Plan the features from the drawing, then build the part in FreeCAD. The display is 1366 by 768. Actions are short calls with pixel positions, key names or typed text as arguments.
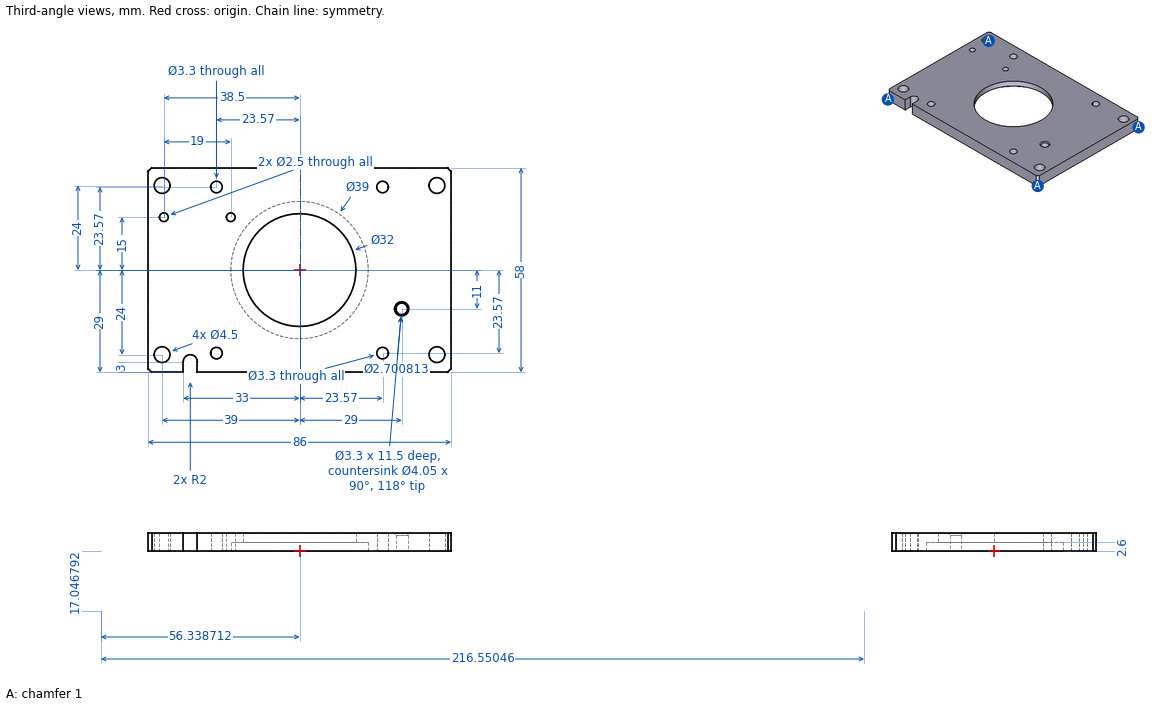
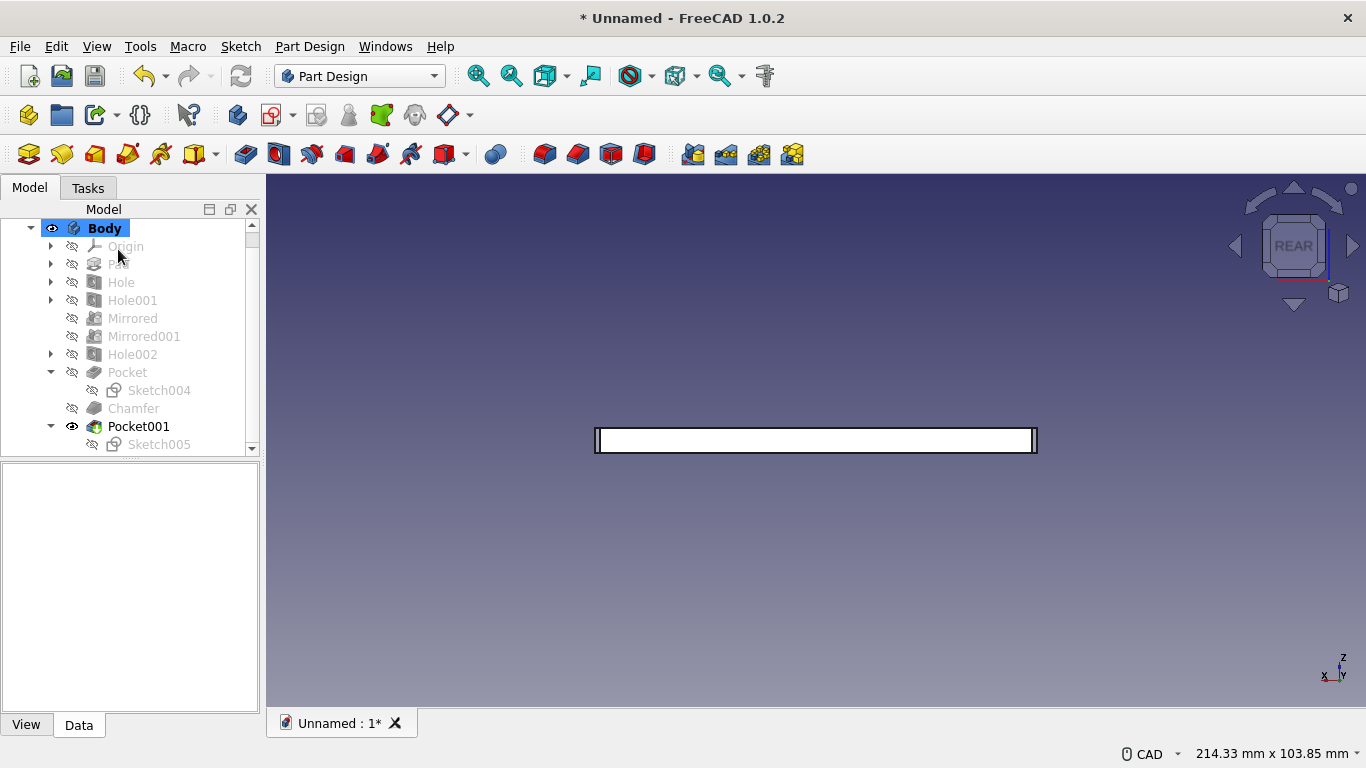
click(270, 116)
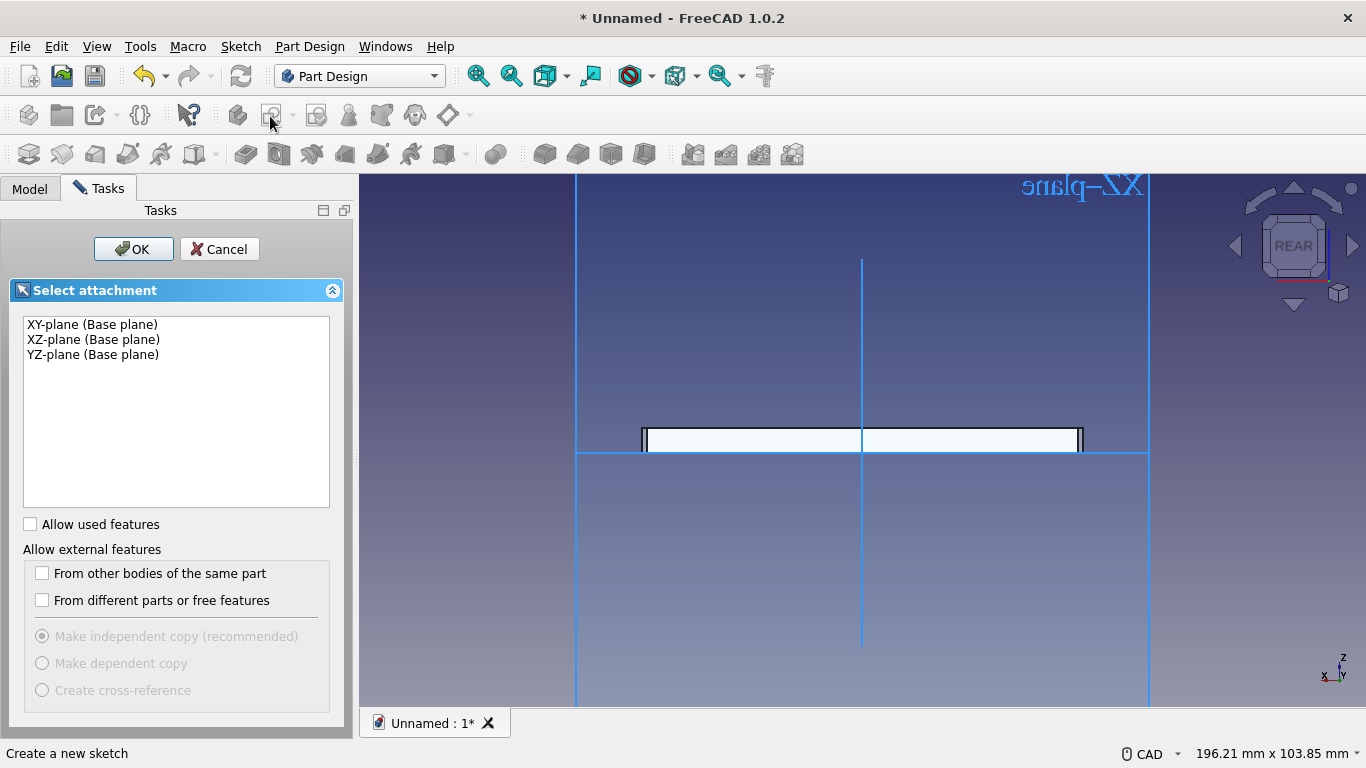
click(84, 324)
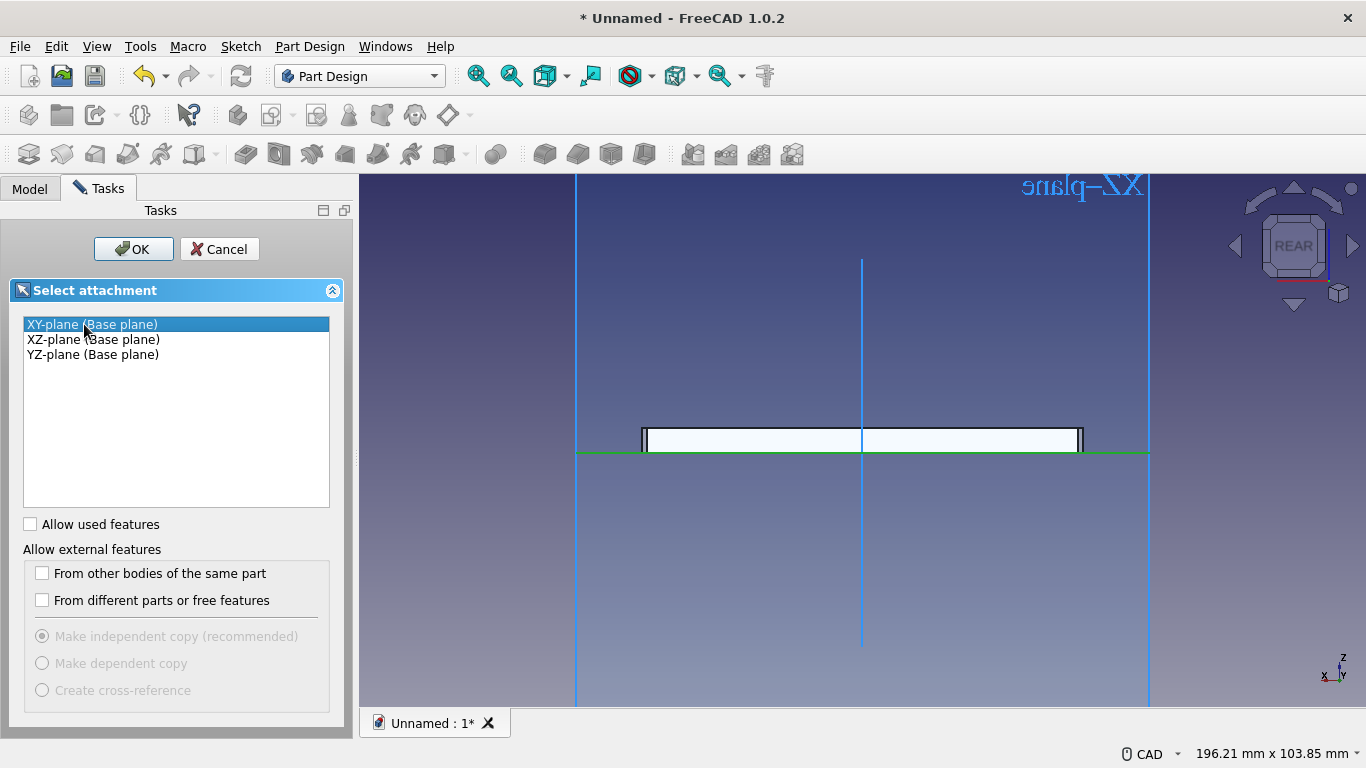
click(134, 249)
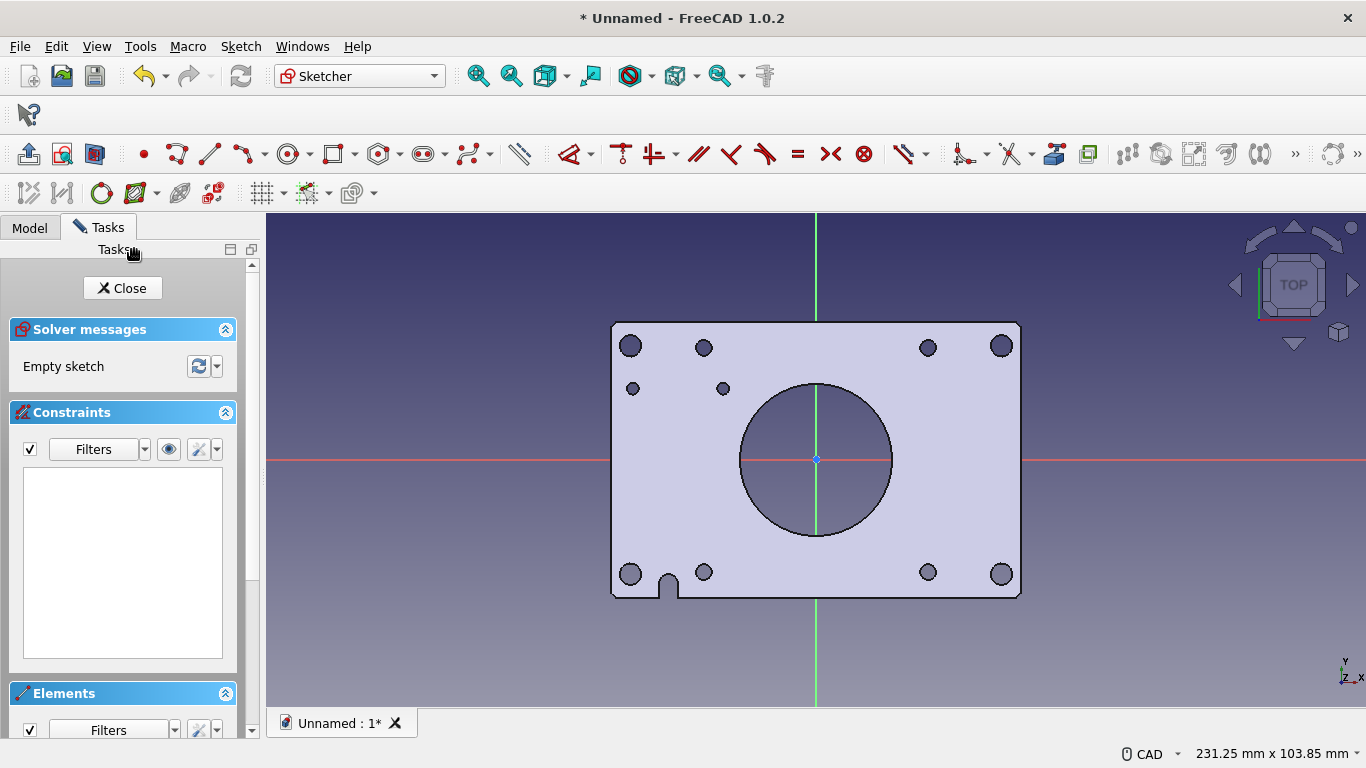
key(q)
key(s)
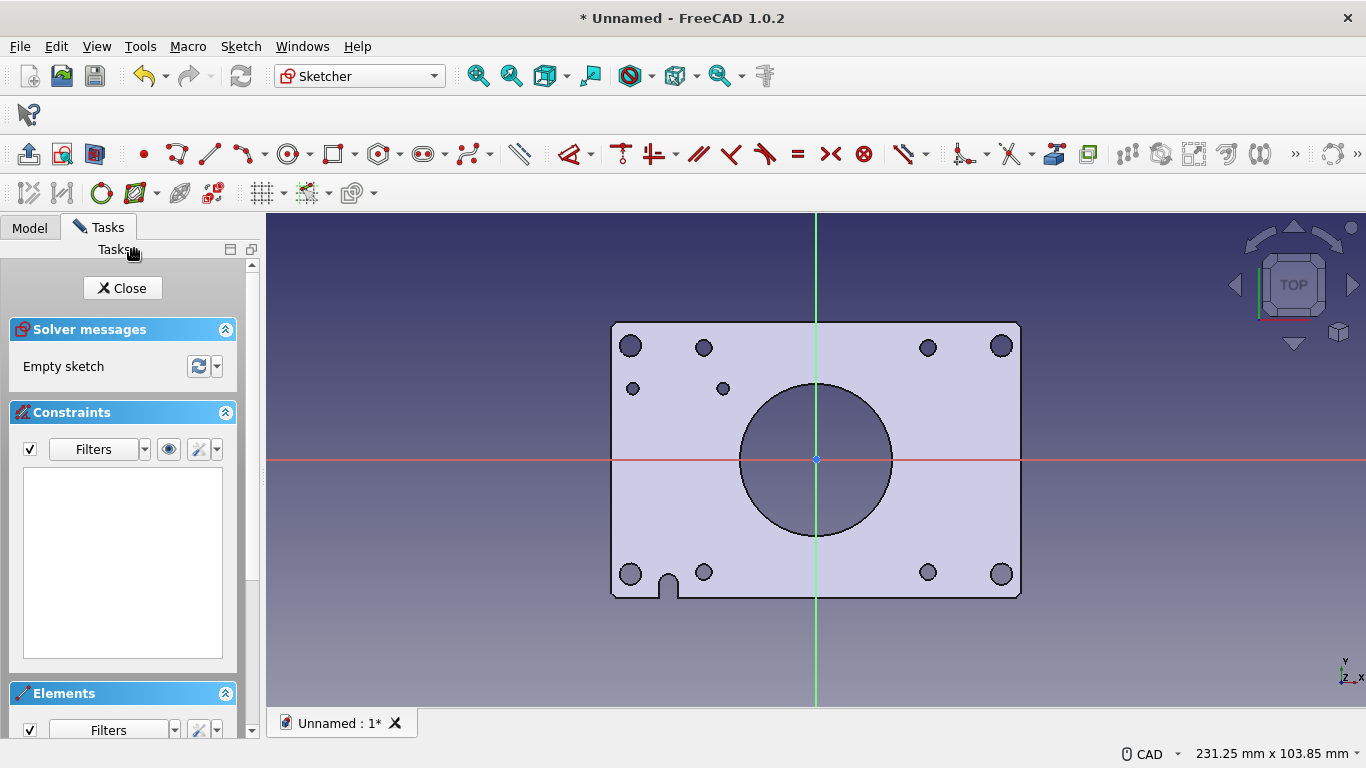
scroll(899, 460, up, 3)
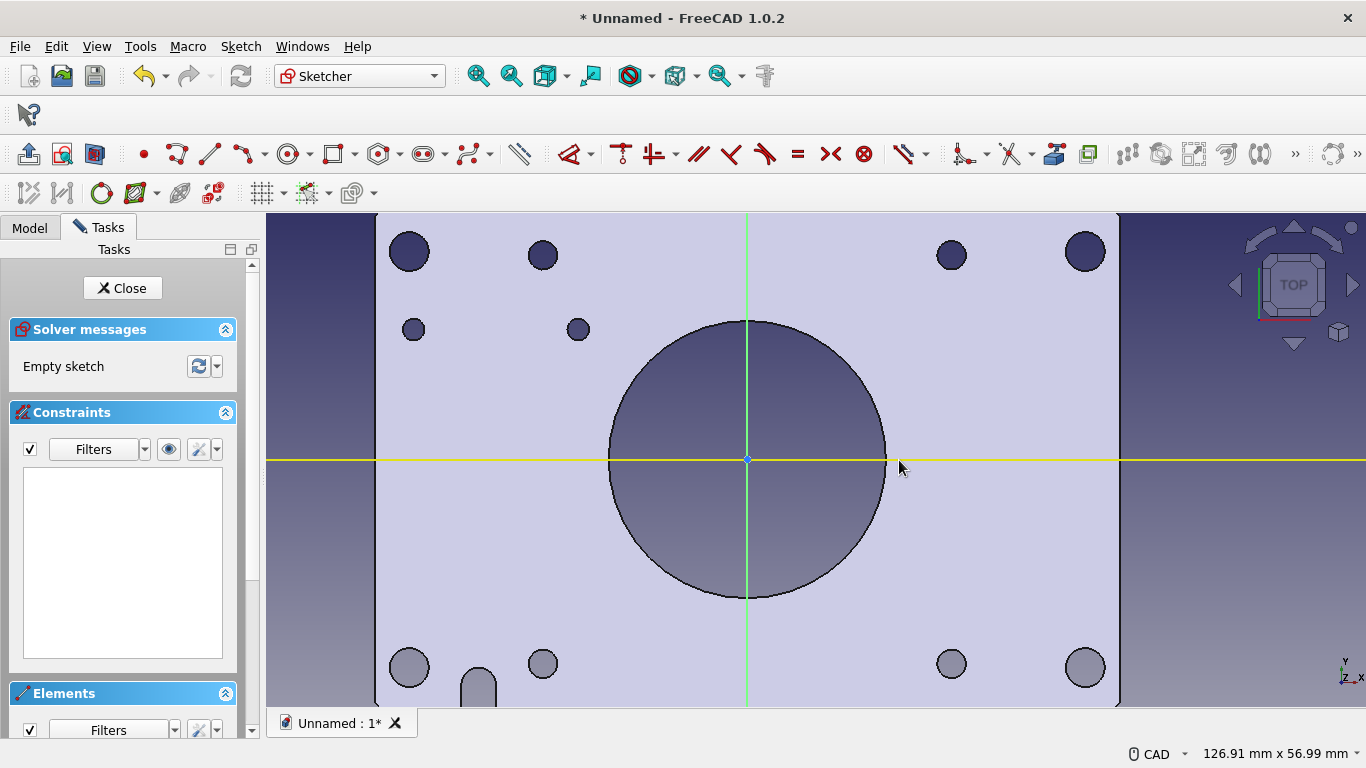
click(288, 154)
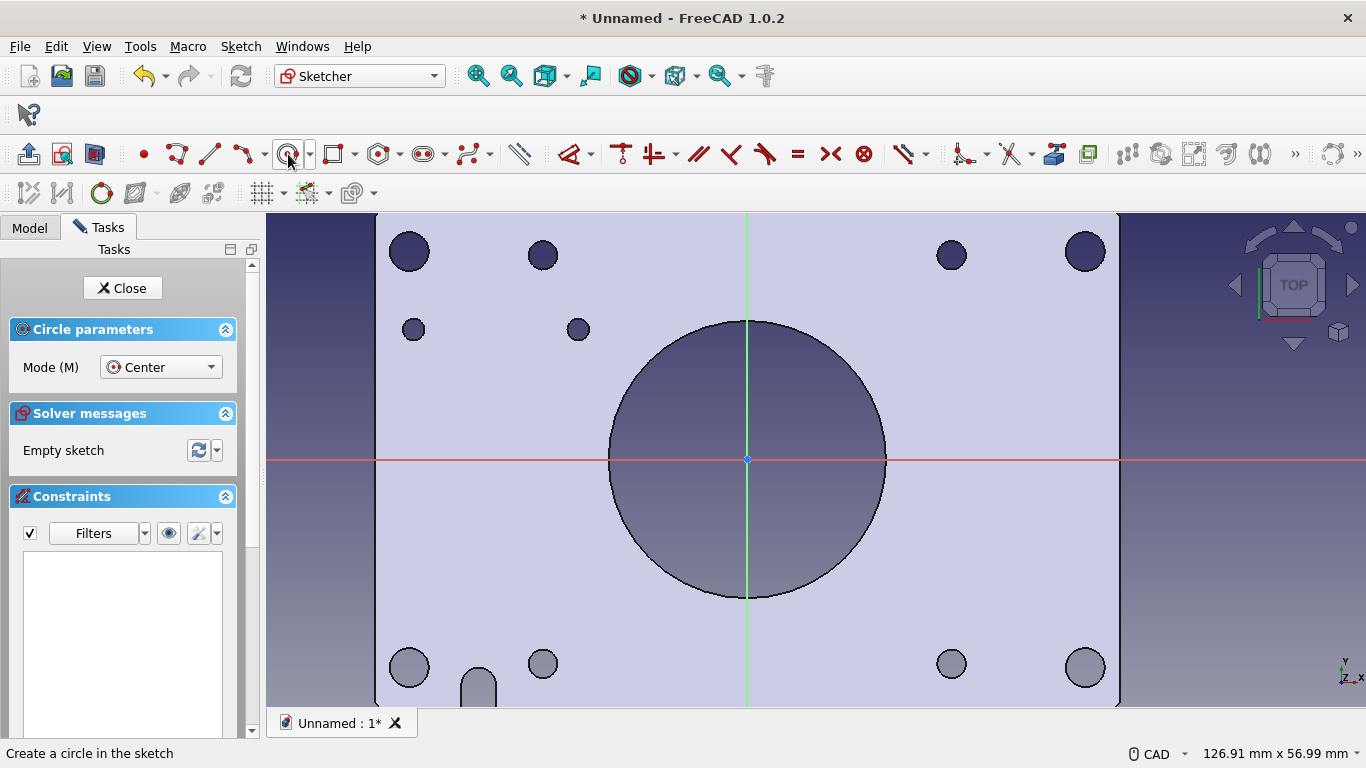
click(747, 460)
move(867, 340)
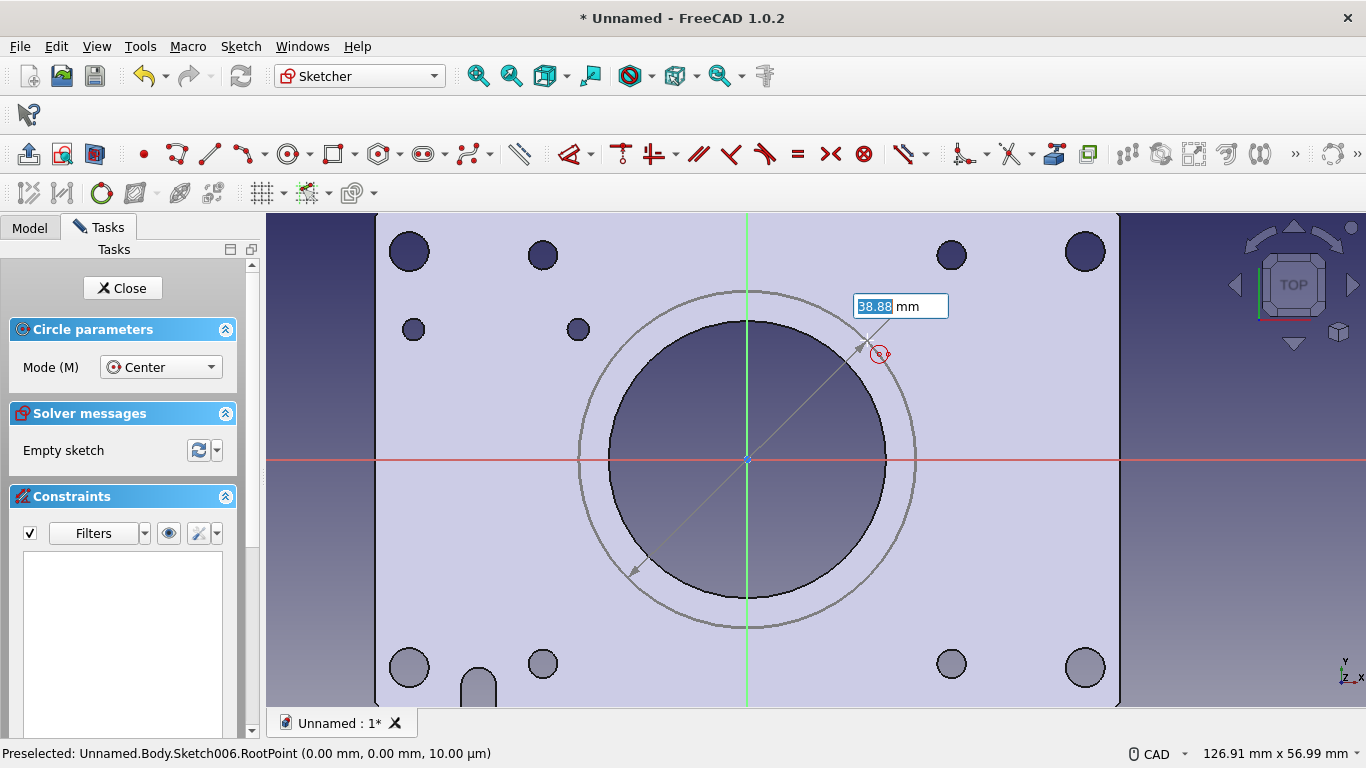
text(39)
key(Return)
key(Escape)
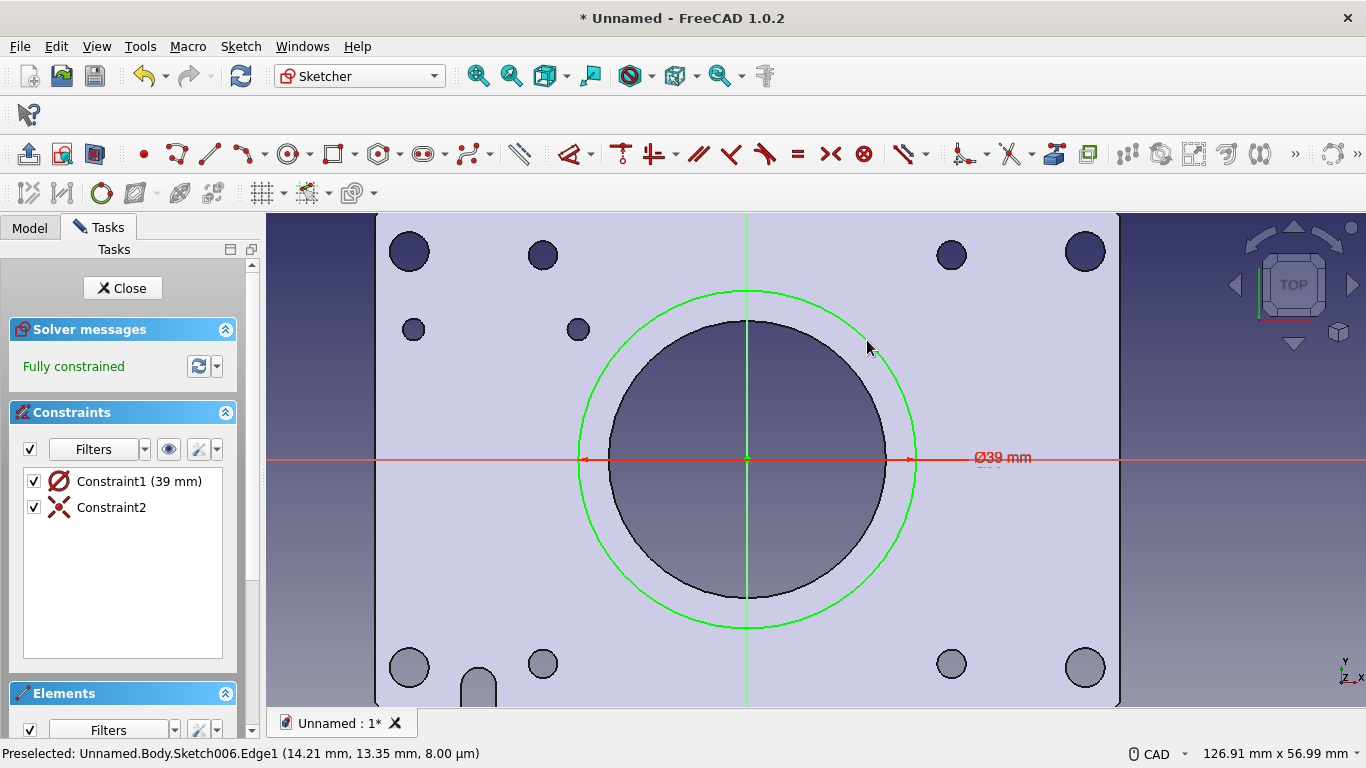
click(123, 288)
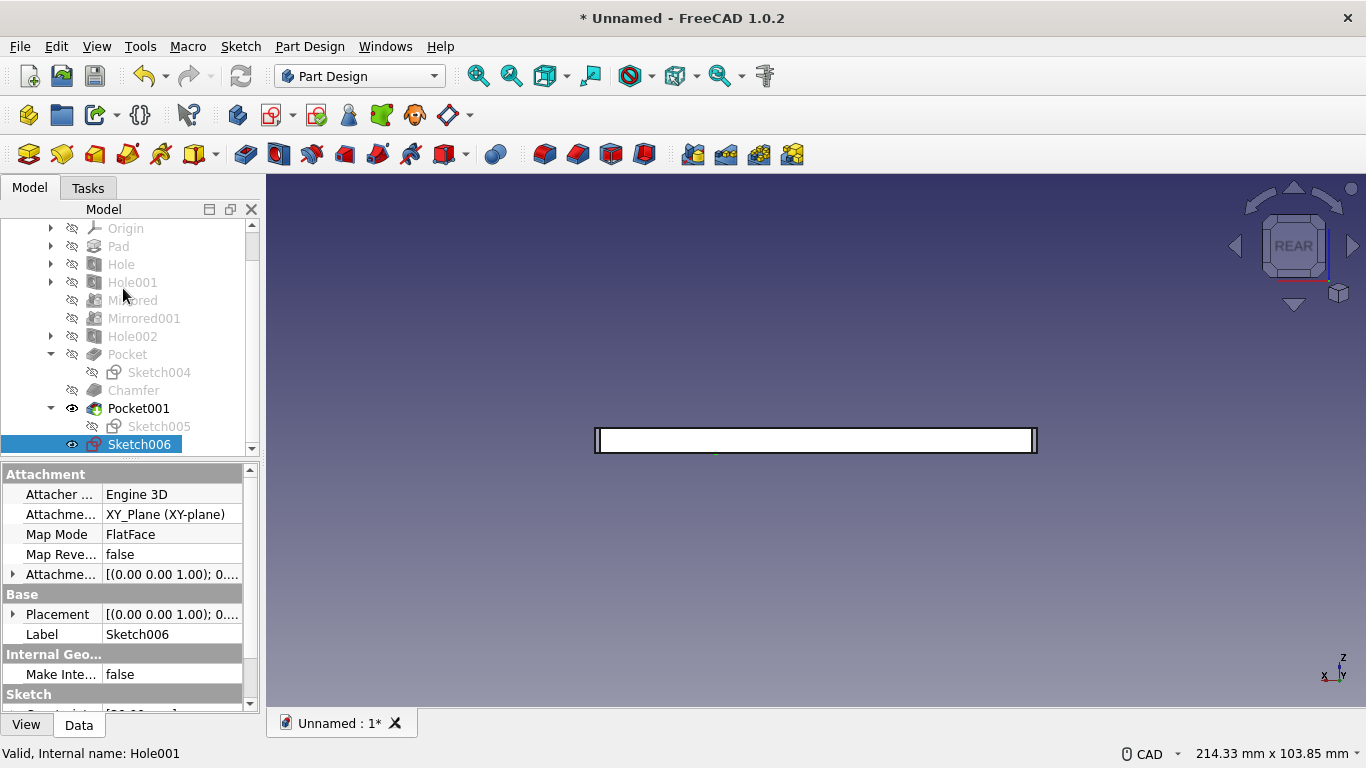
click(246, 154)